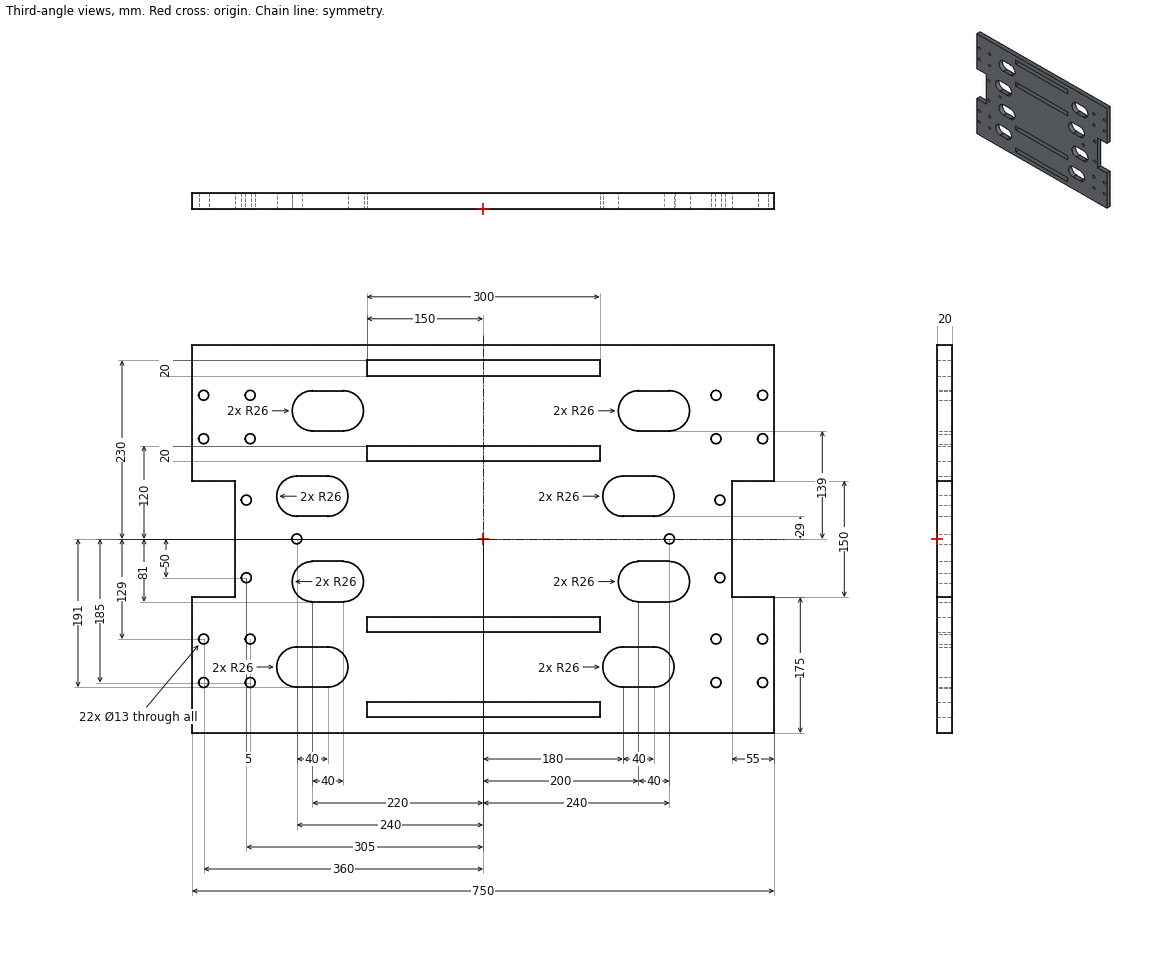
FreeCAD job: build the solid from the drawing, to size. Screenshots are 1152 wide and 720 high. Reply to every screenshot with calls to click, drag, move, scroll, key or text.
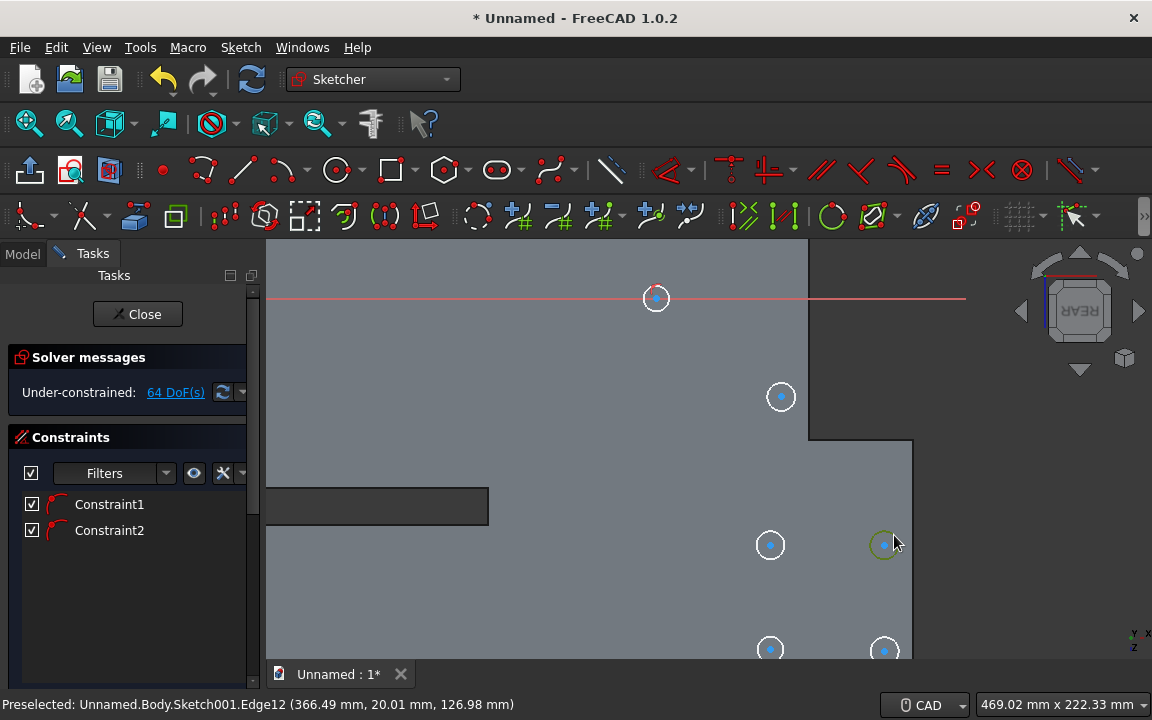
click(780, 535)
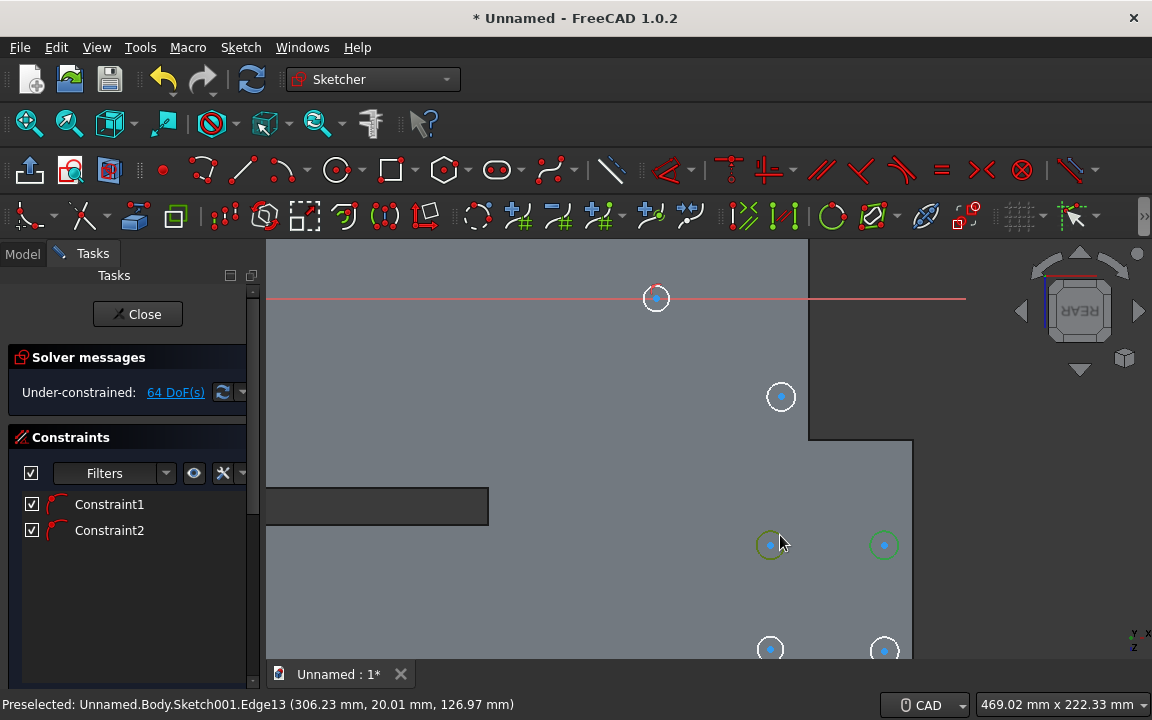
scroll(894, 536, down, 5)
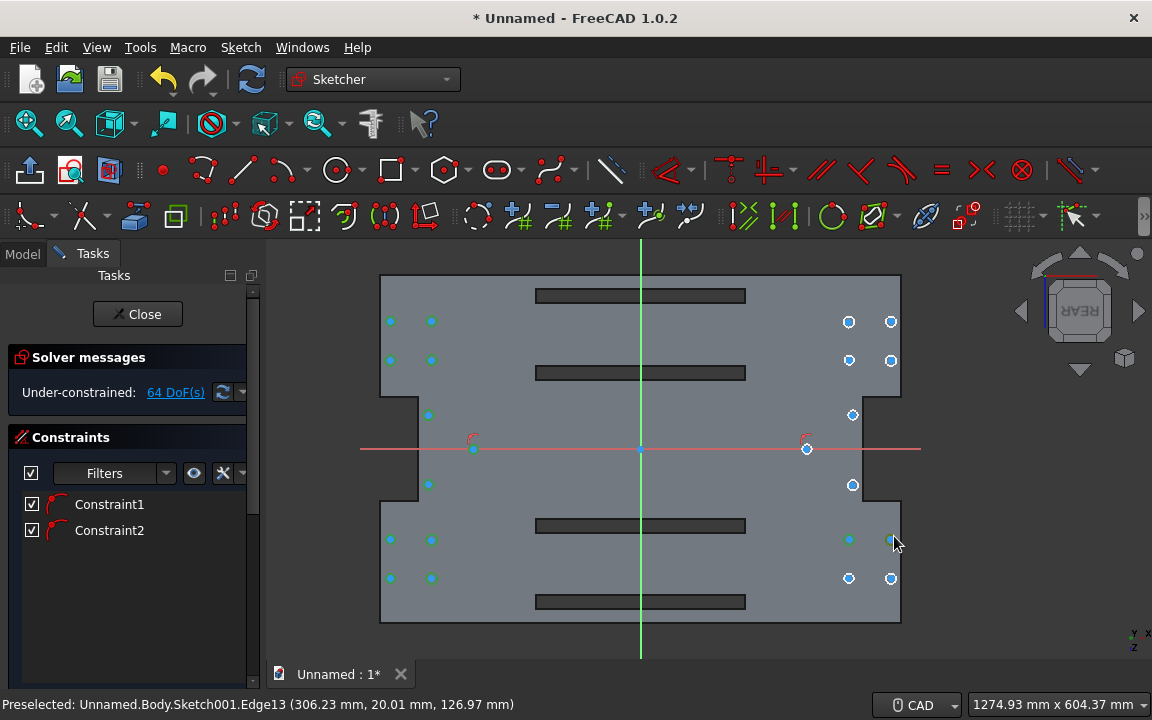
scroll(895, 575, up, 5)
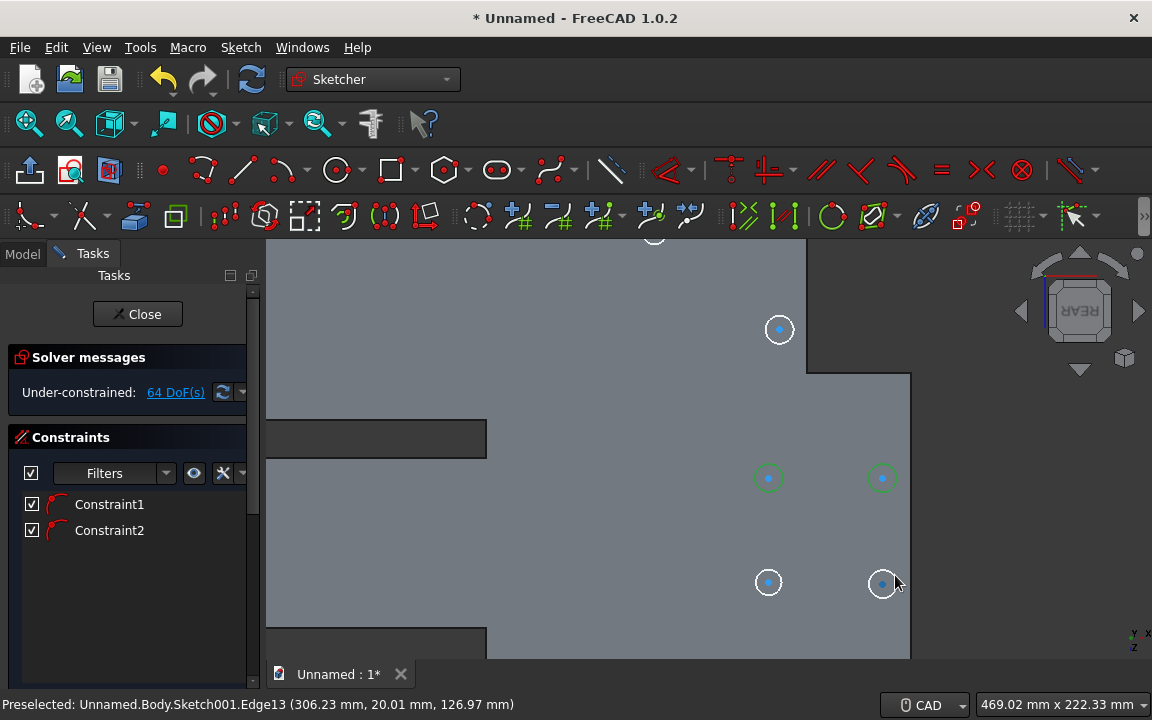
click(893, 574)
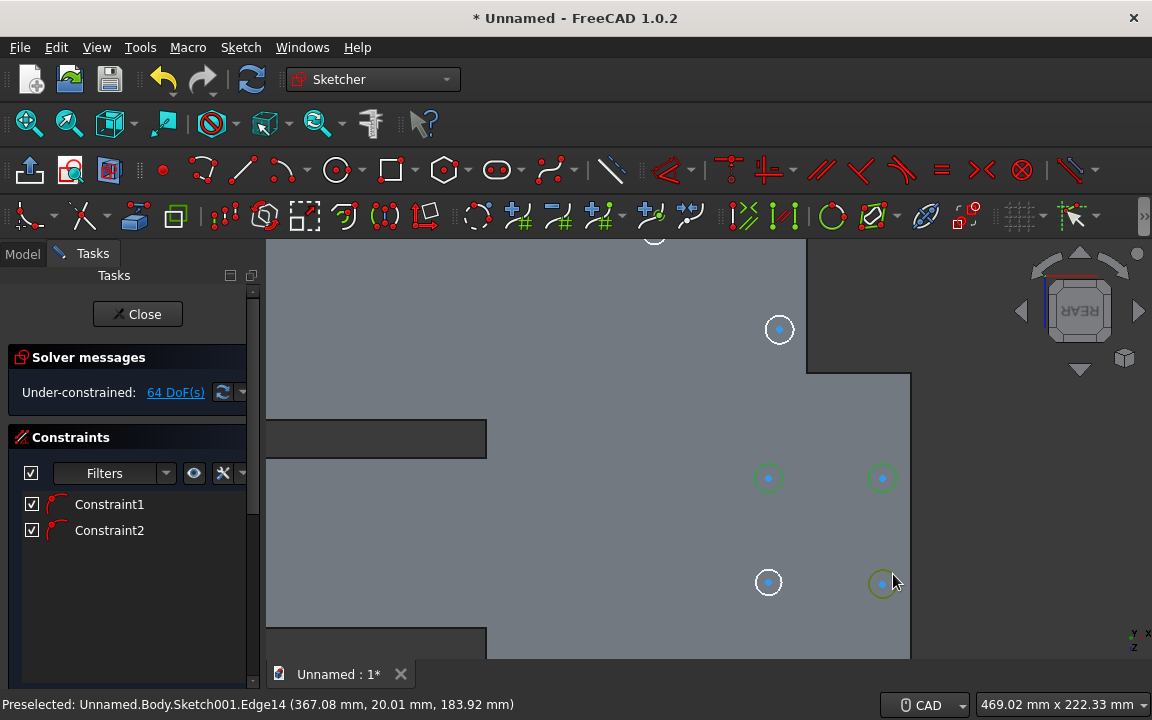
scroll(895, 576, down, 5)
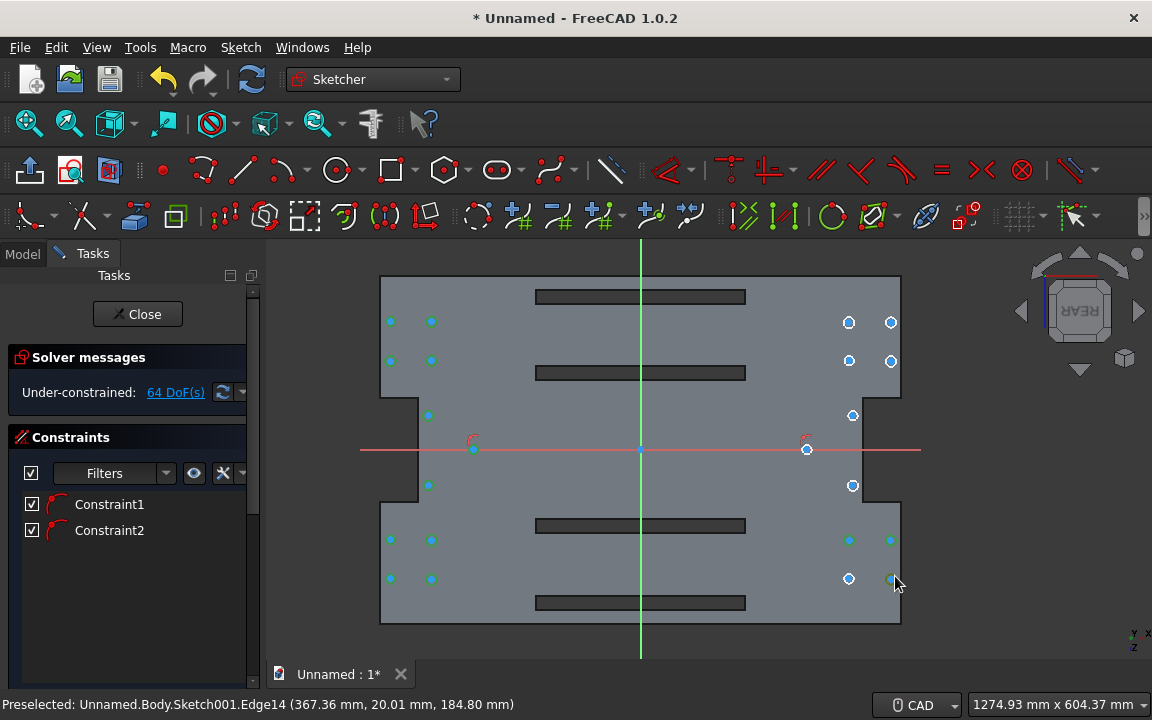
scroll(895, 358, up, 5)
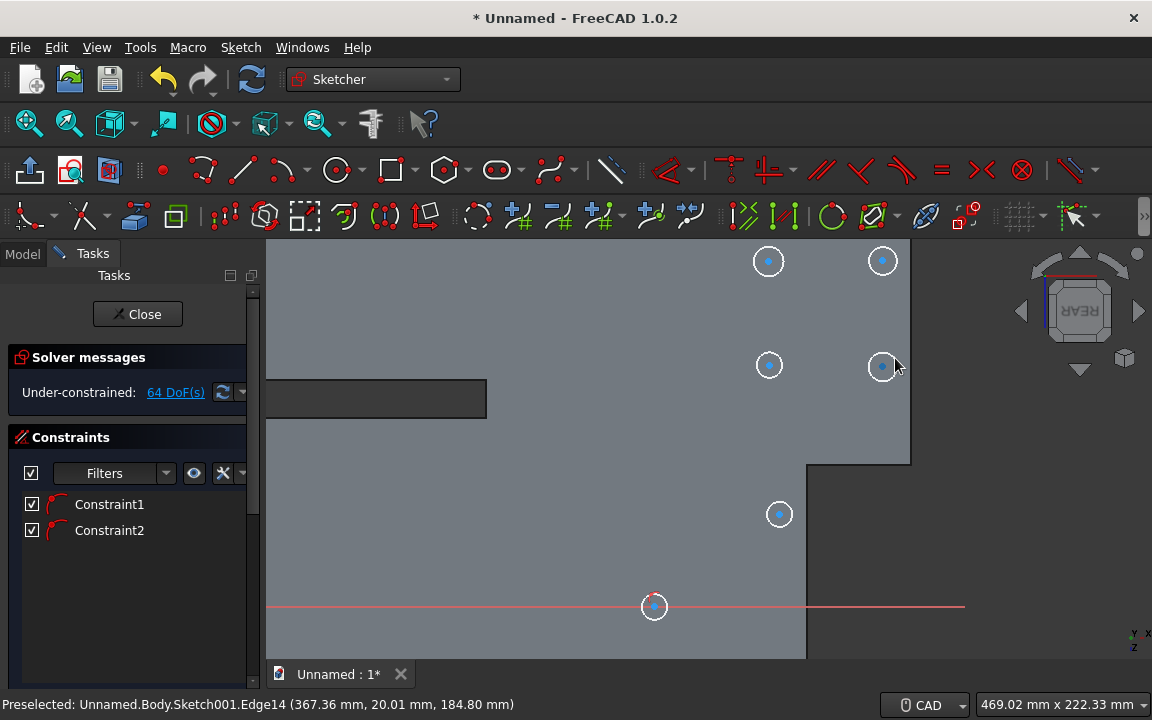
click(893, 357)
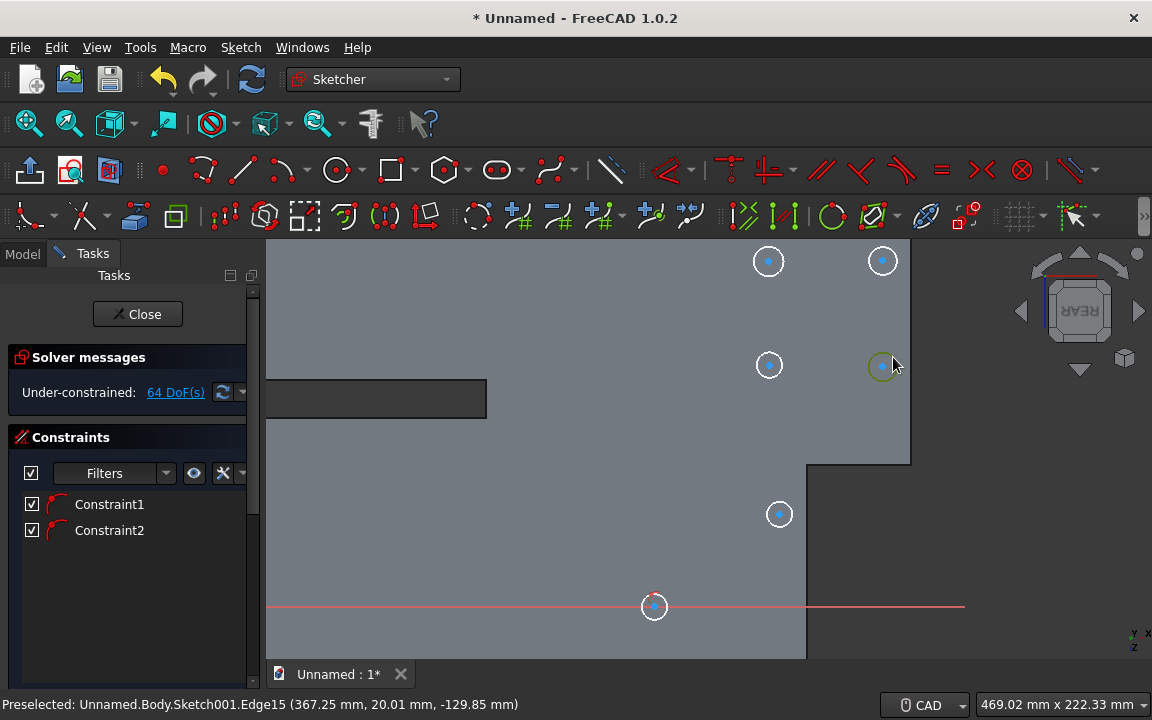
click(873, 271)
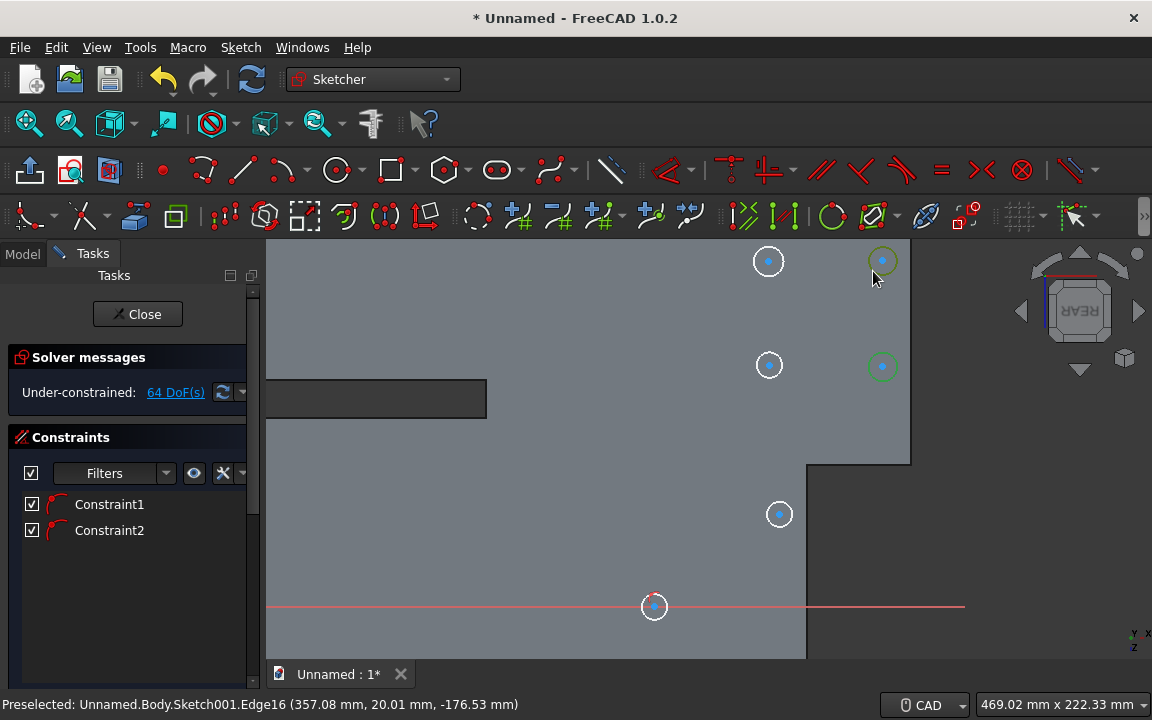
click(778, 356)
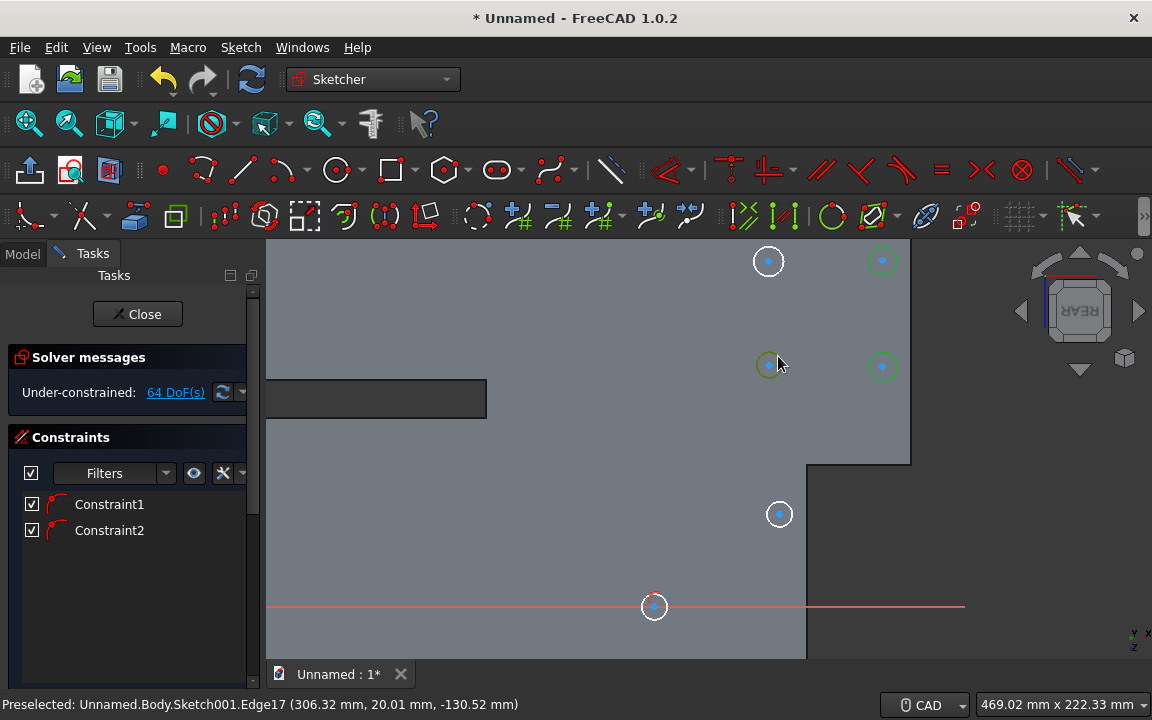
scroll(895, 357, down, 5)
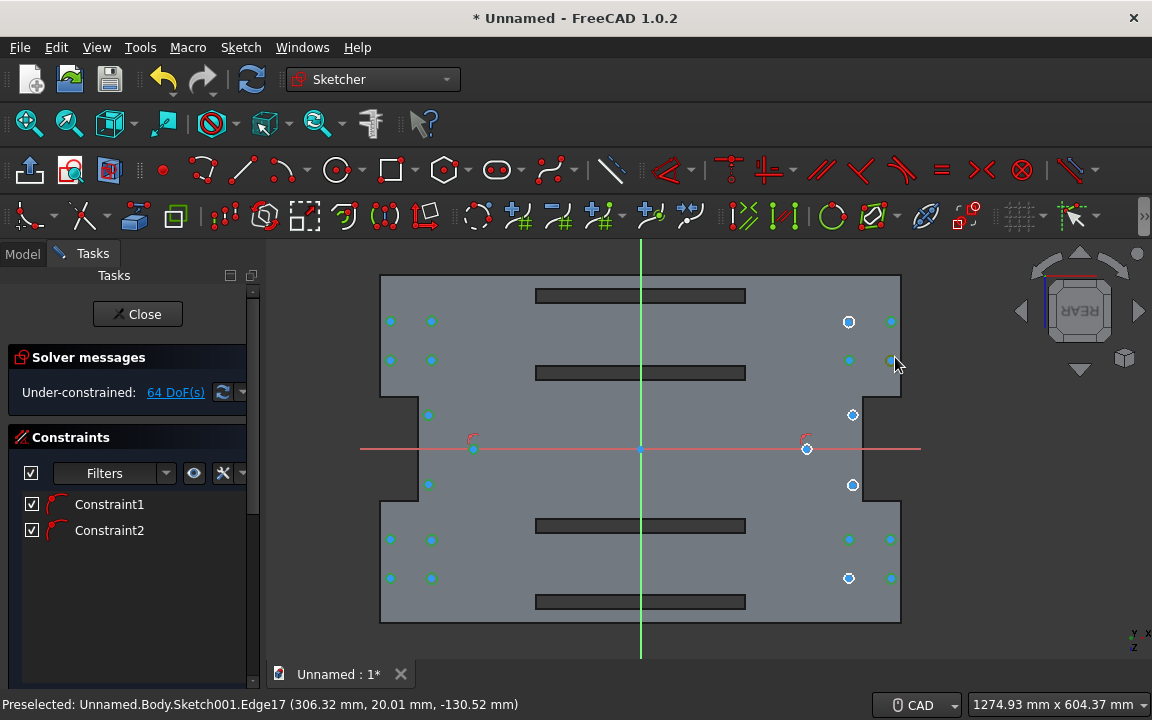
scroll(857, 482, up, 5)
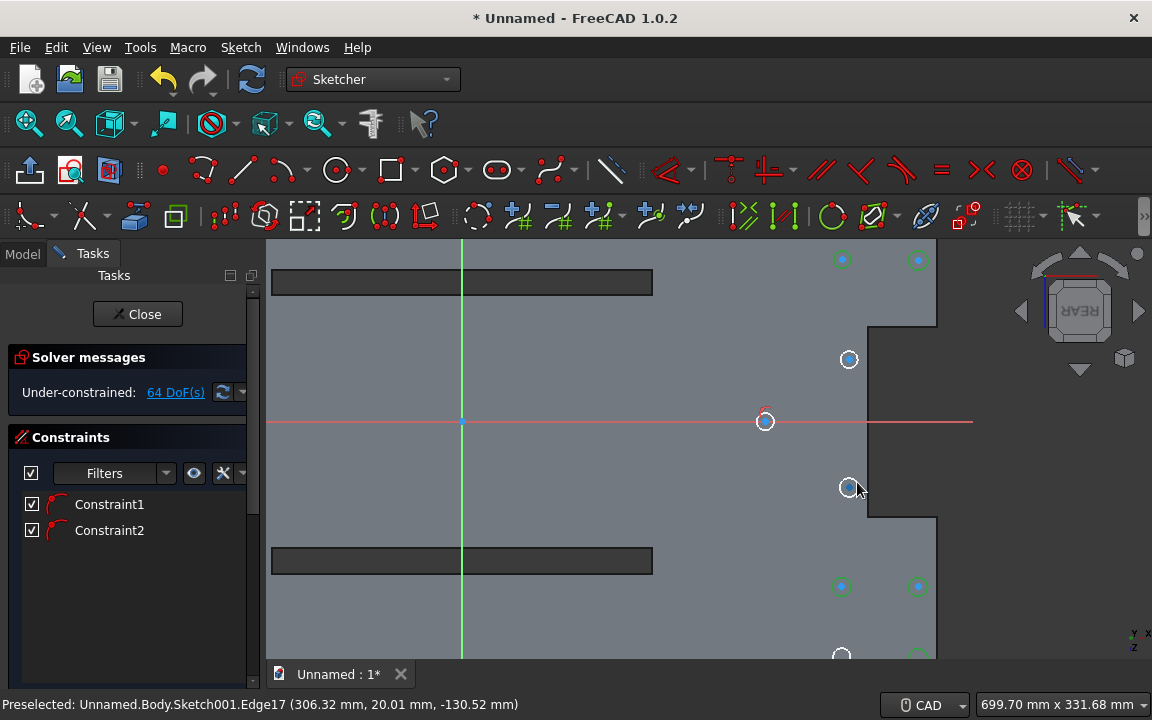
click(855, 480)